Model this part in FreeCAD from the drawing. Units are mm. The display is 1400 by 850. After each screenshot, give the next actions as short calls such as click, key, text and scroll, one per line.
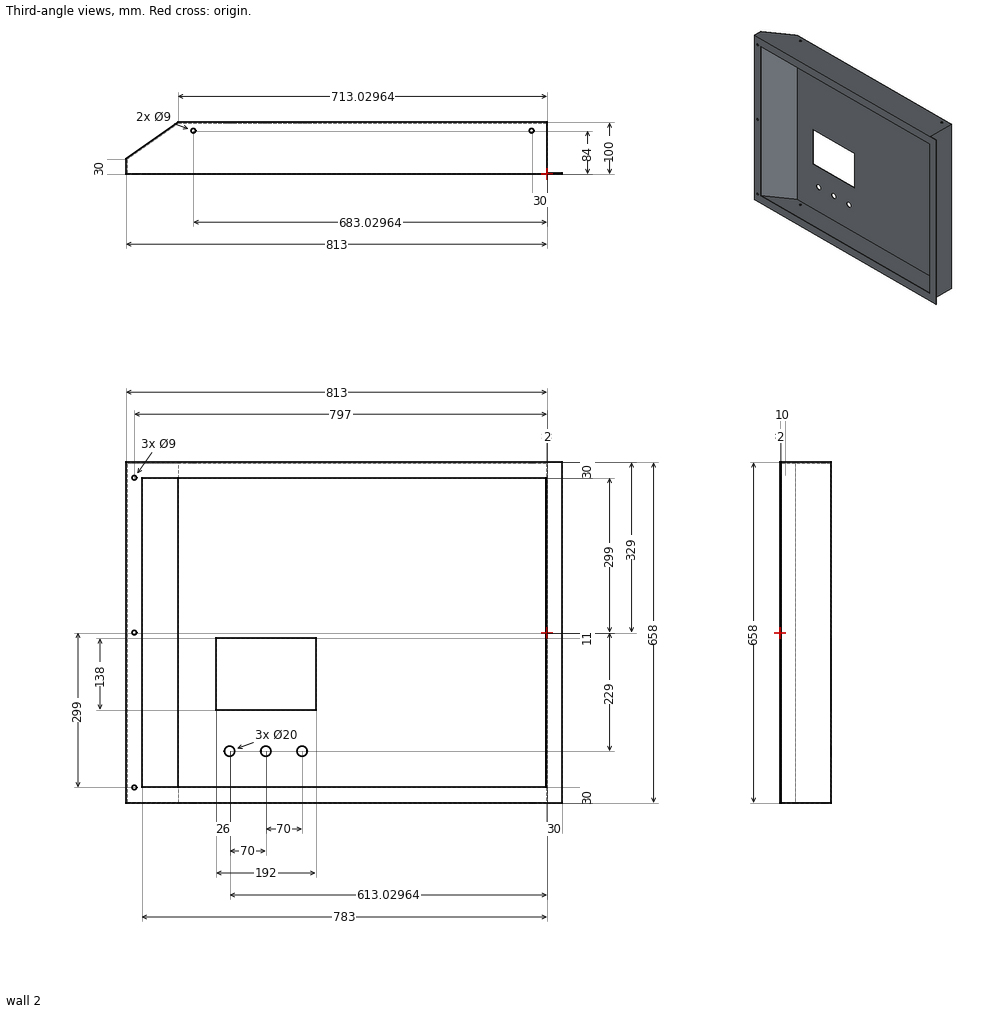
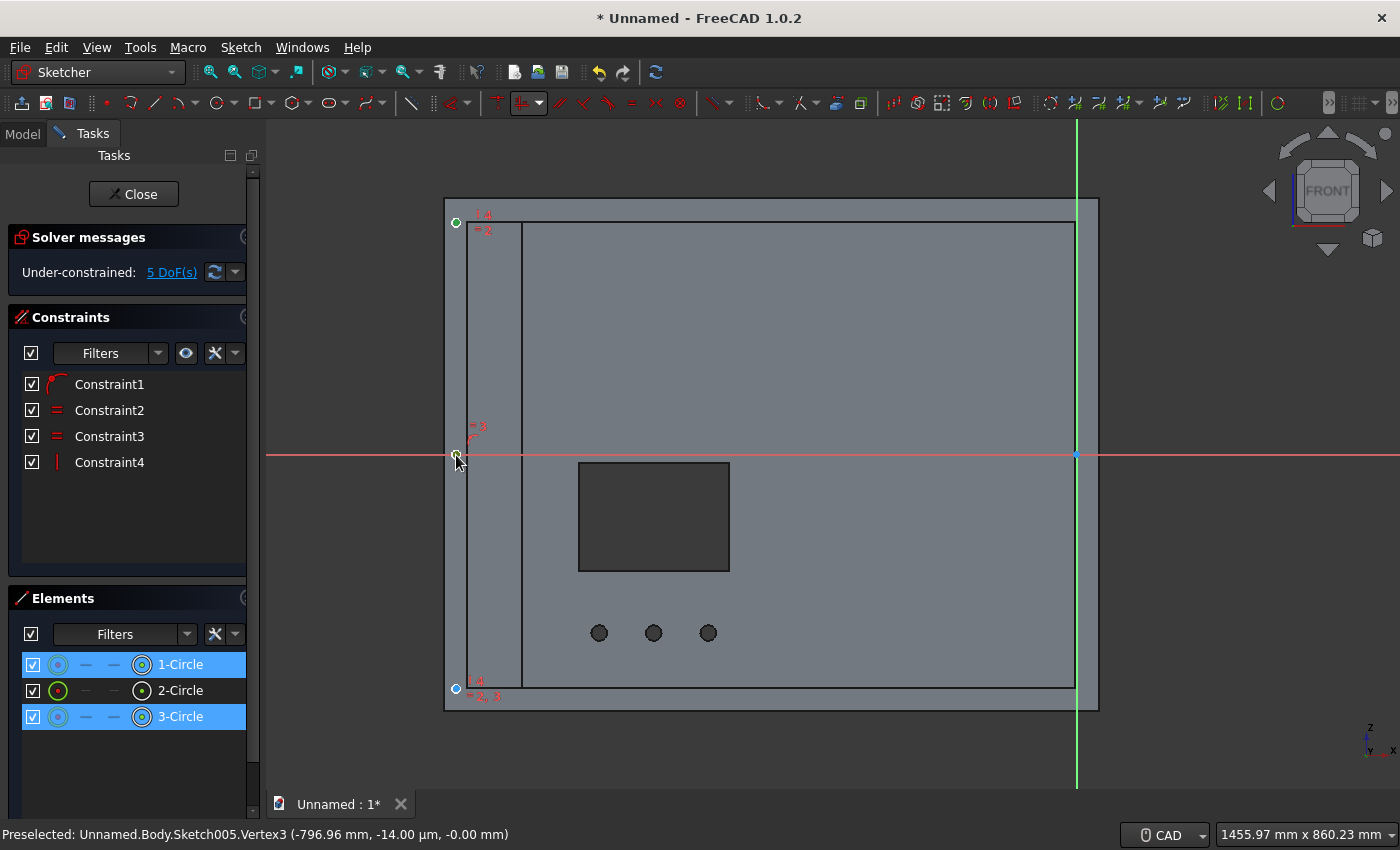
click(542, 104)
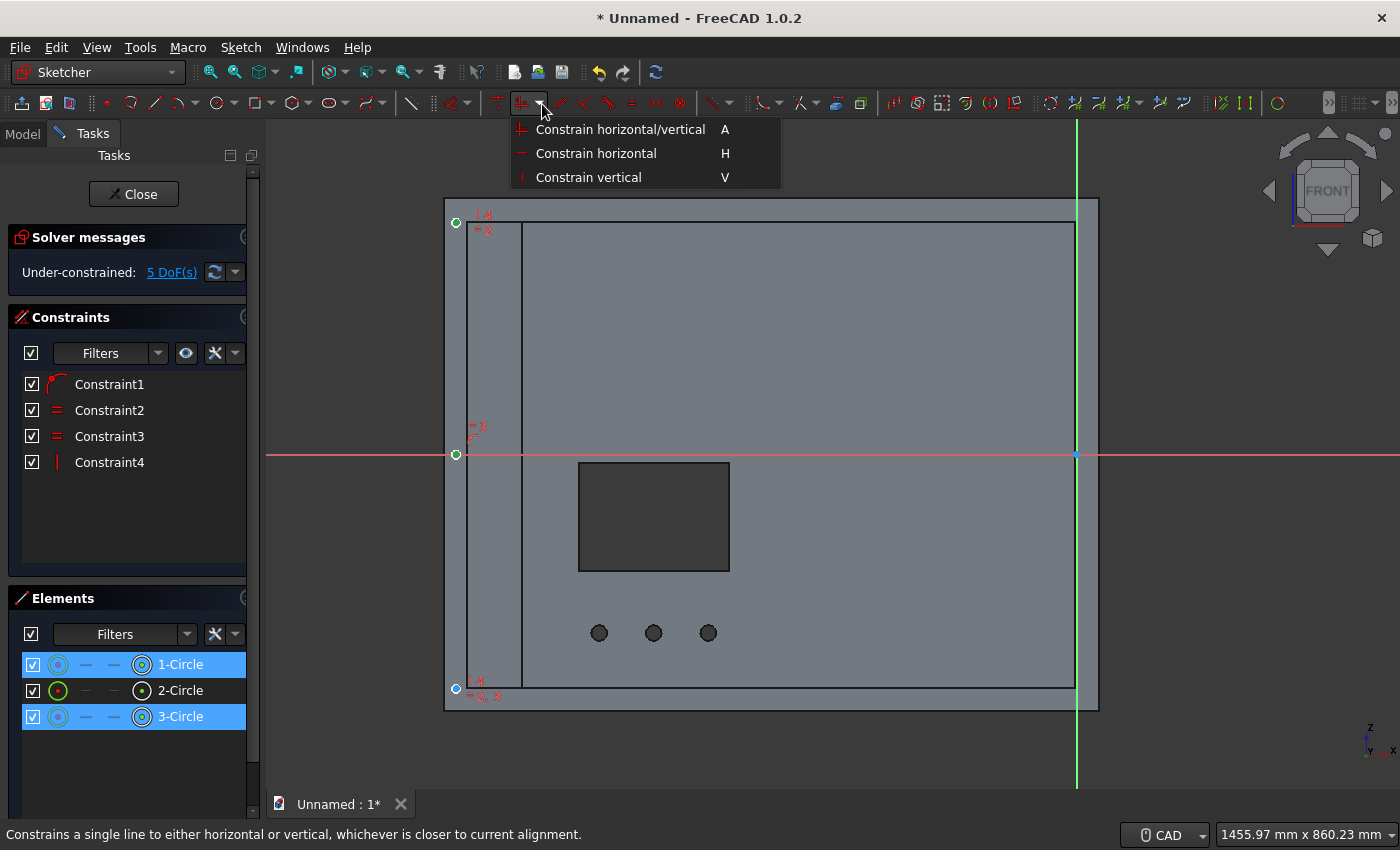
click(646, 177)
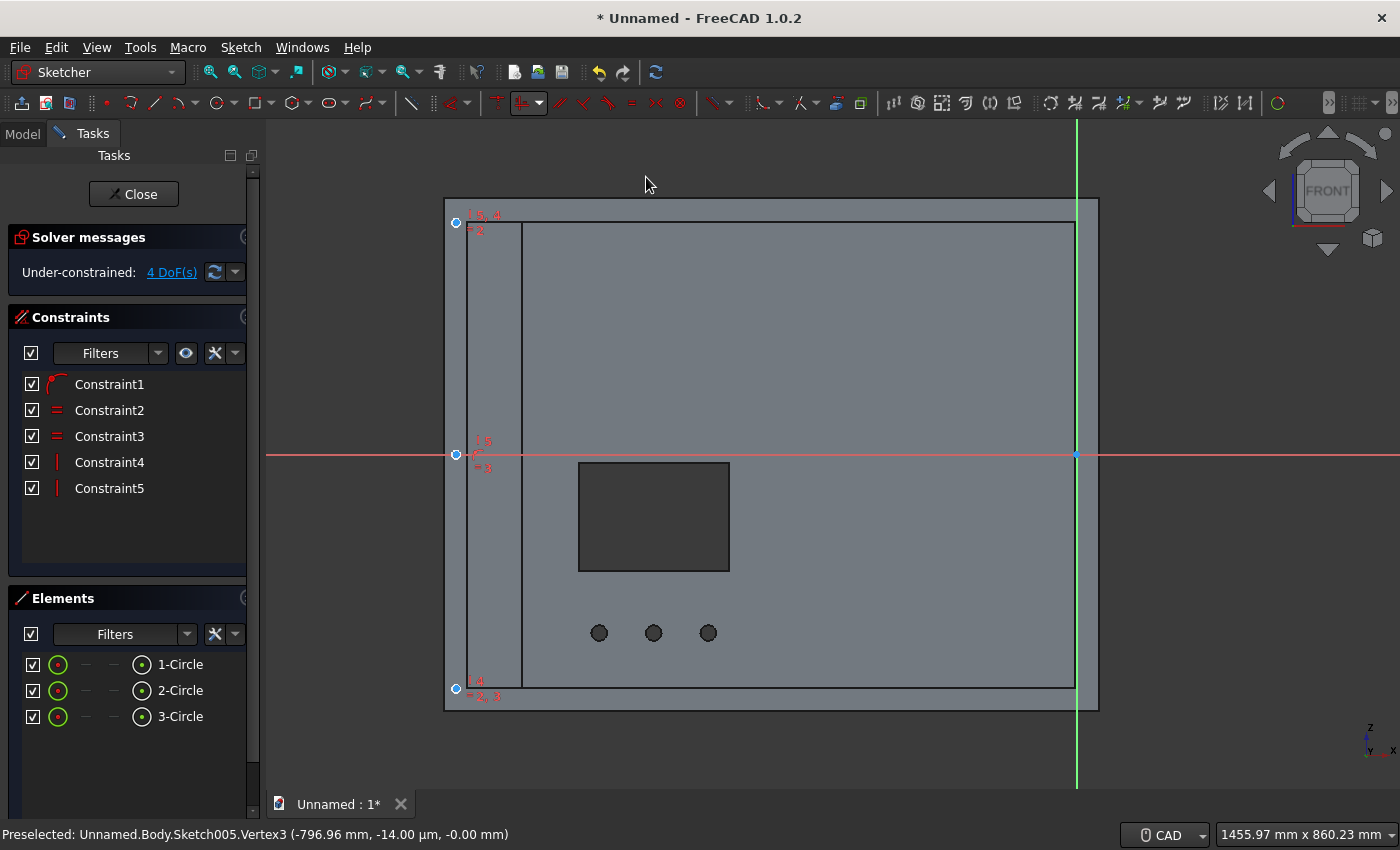
click(450, 104)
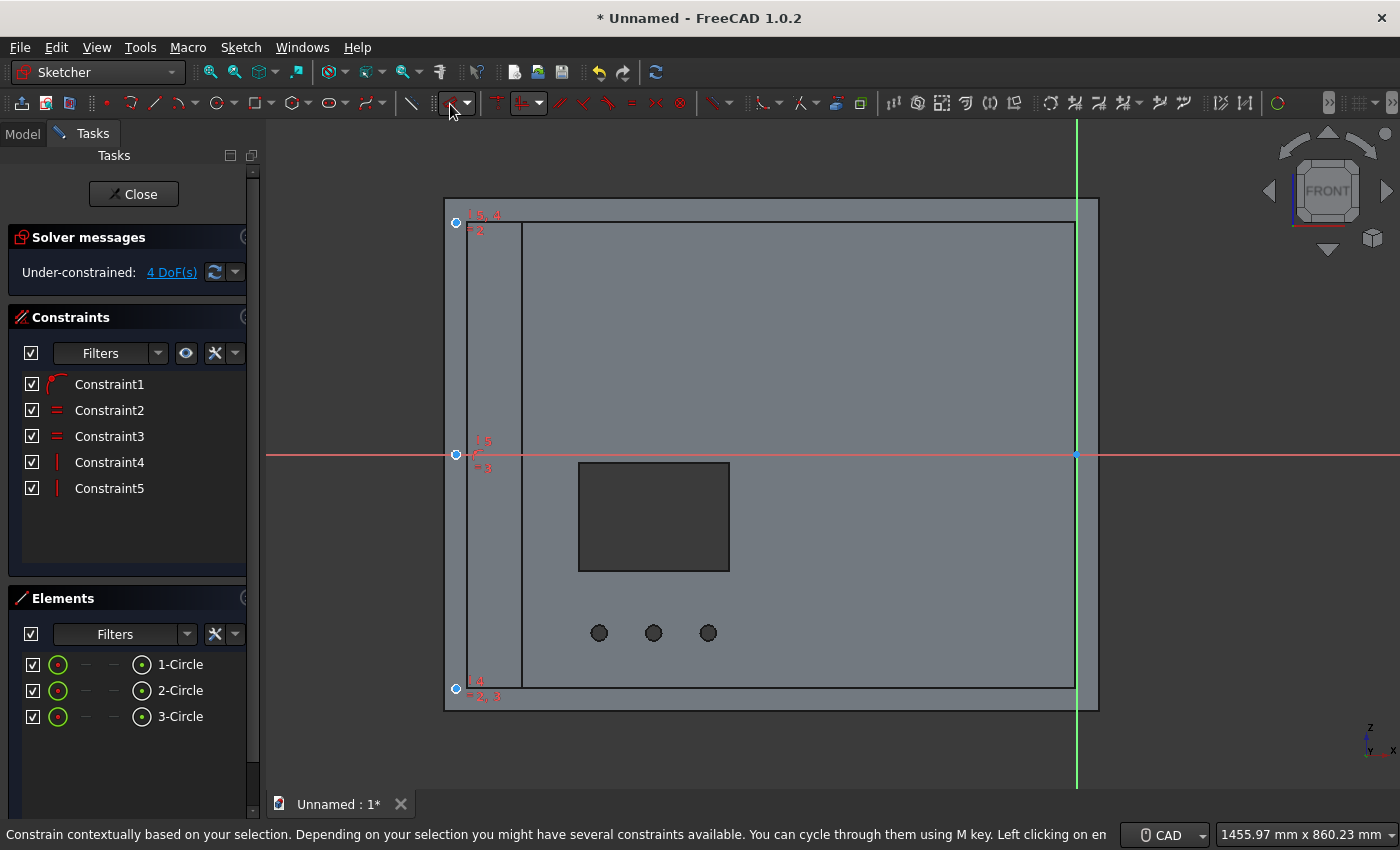
scroll(456, 219, up, 9)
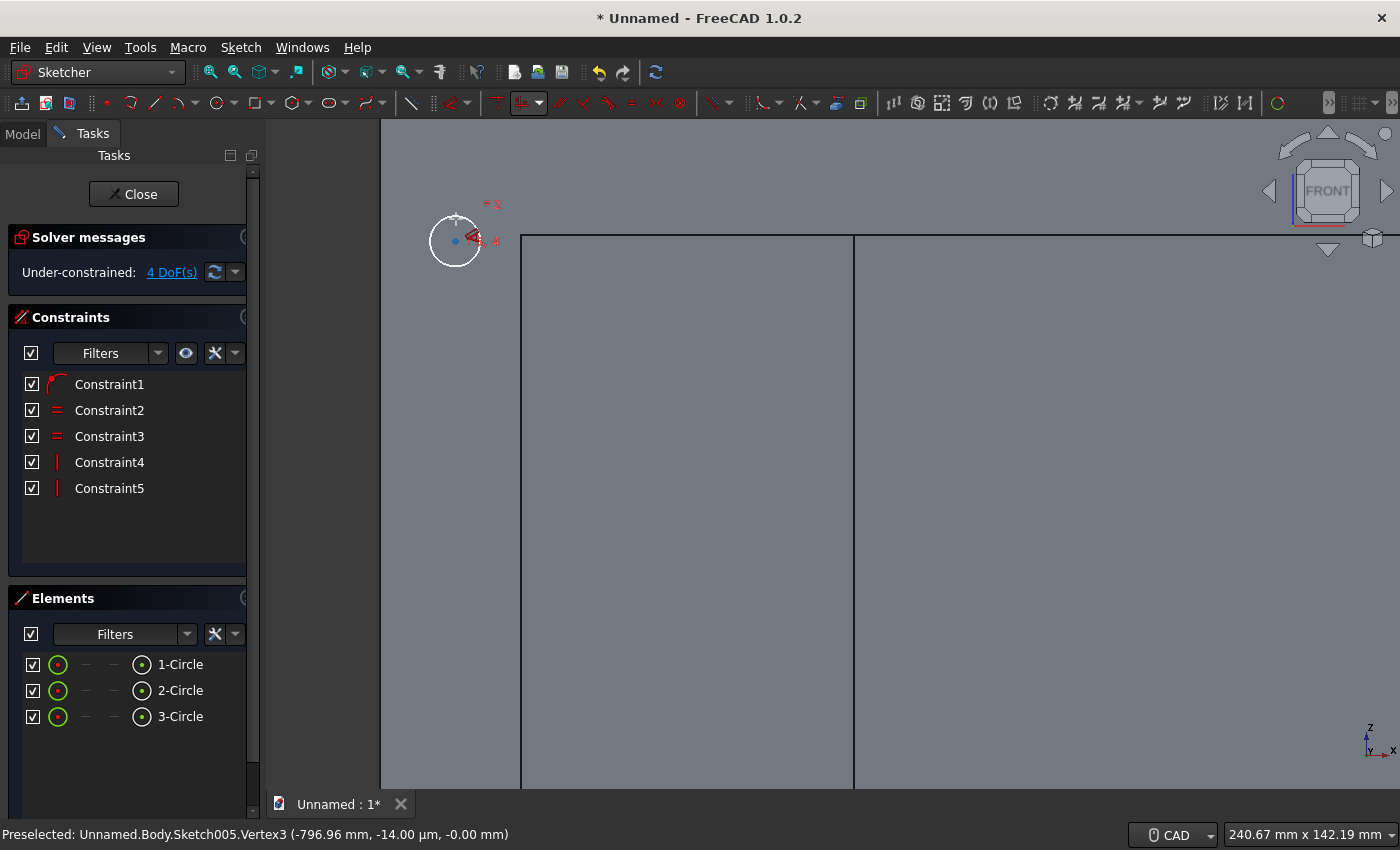
click(456, 216)
click(457, 184)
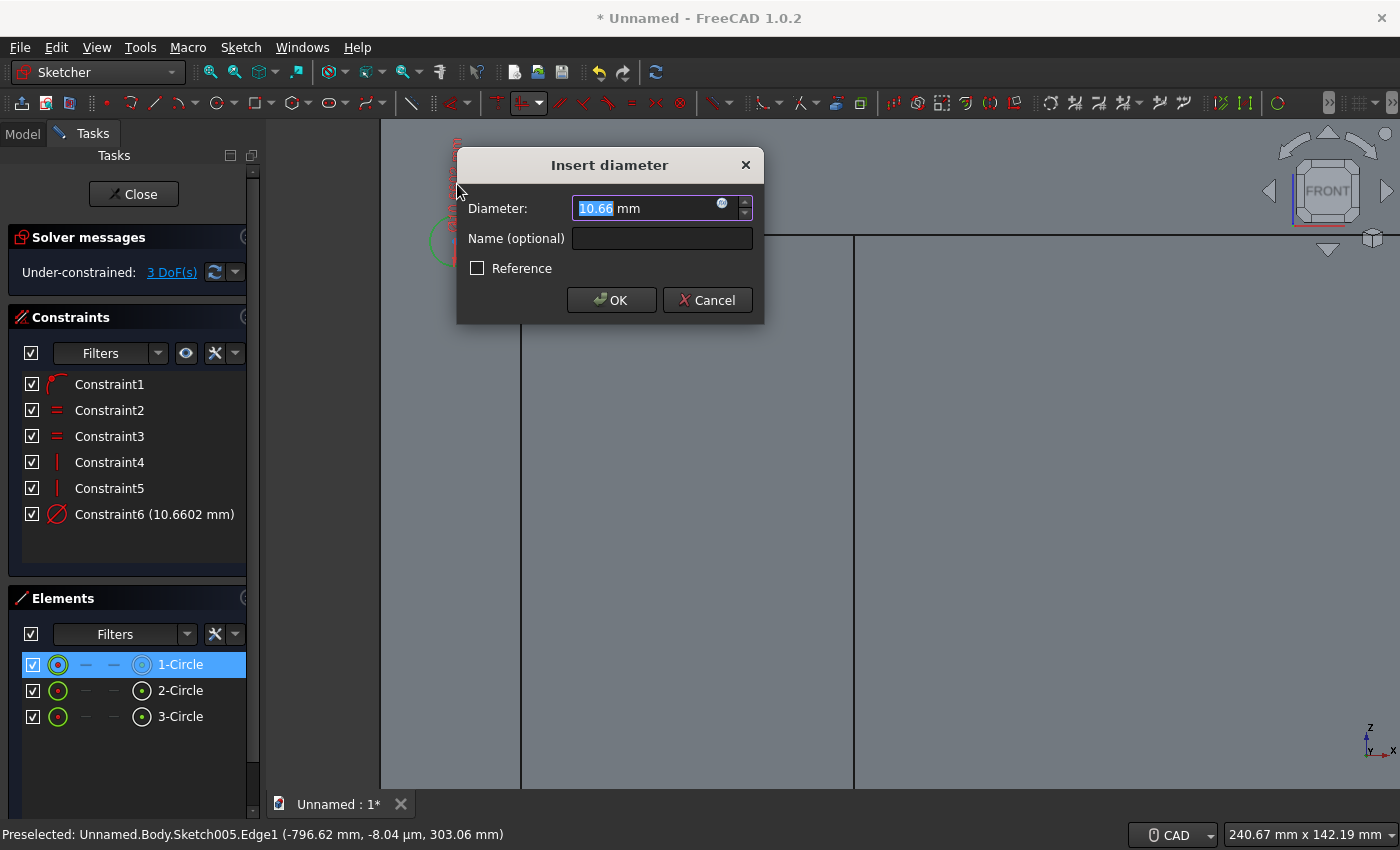
text(9)
key(Return)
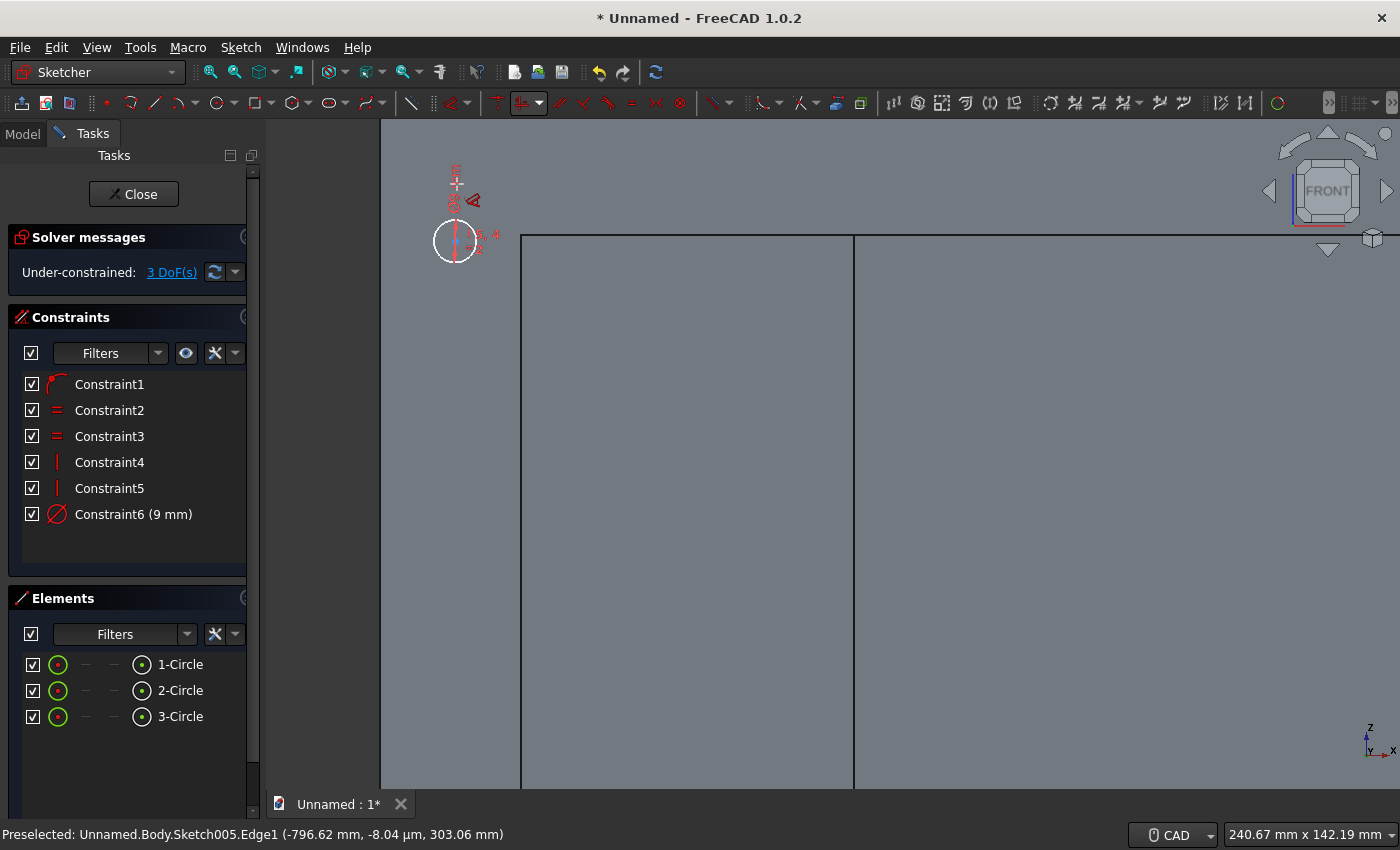
scroll(456, 218, down, 9)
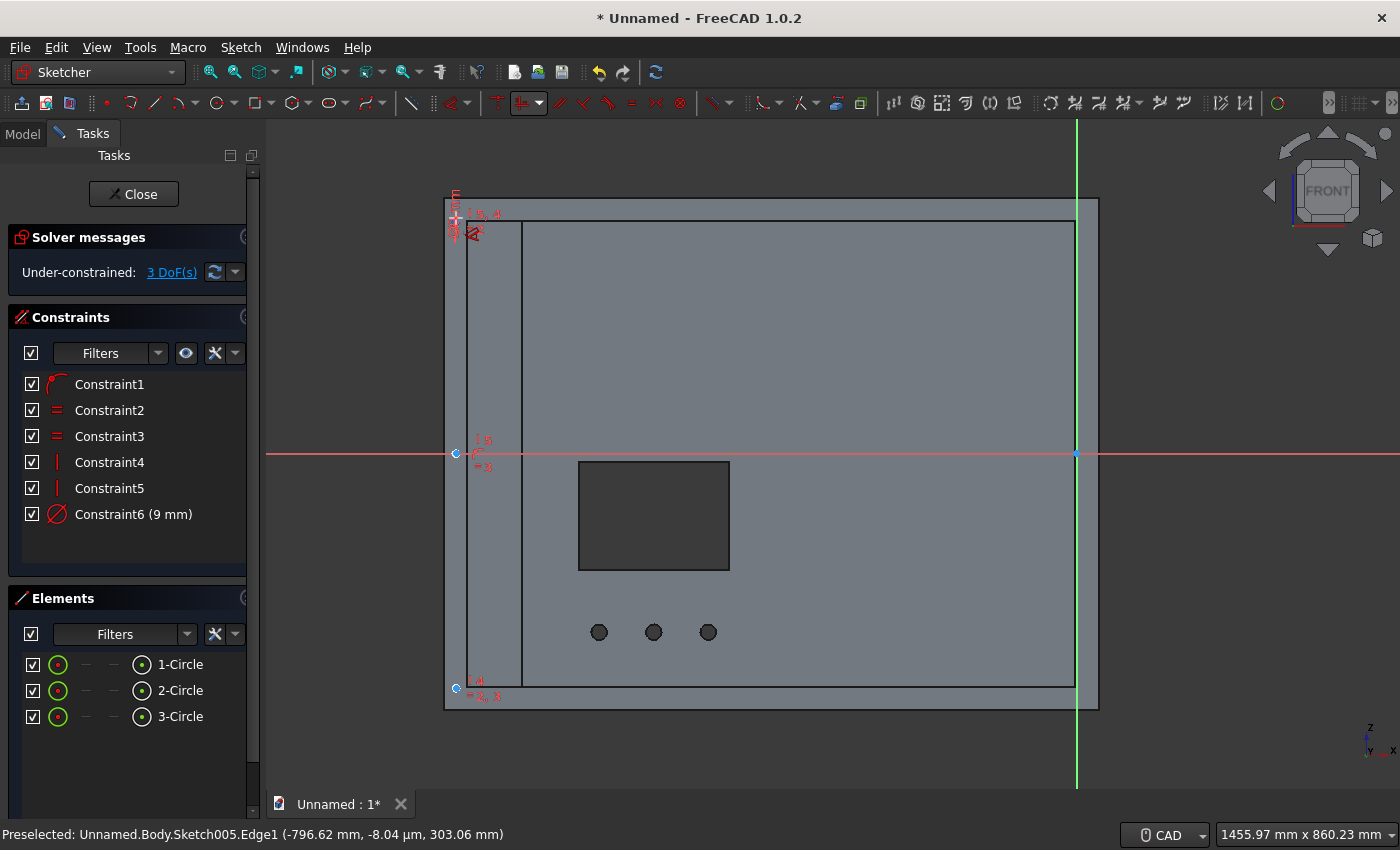
click(456, 222)
click(766, 188)